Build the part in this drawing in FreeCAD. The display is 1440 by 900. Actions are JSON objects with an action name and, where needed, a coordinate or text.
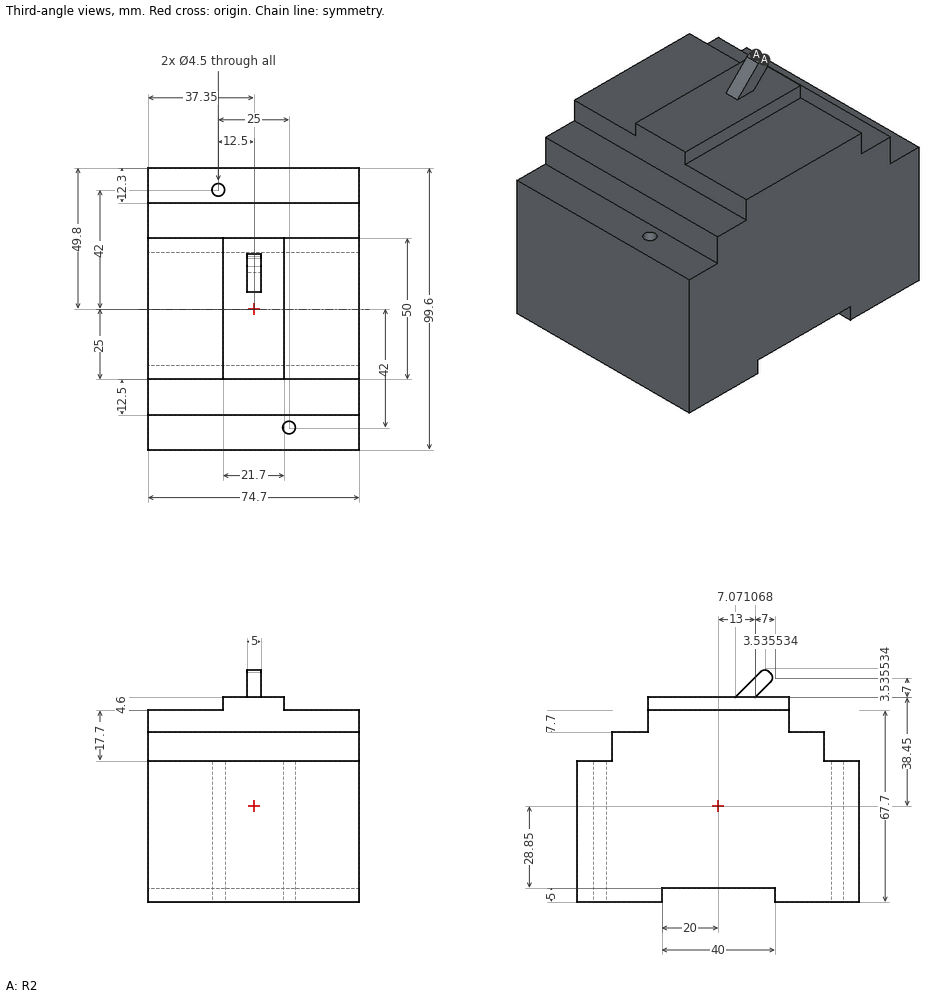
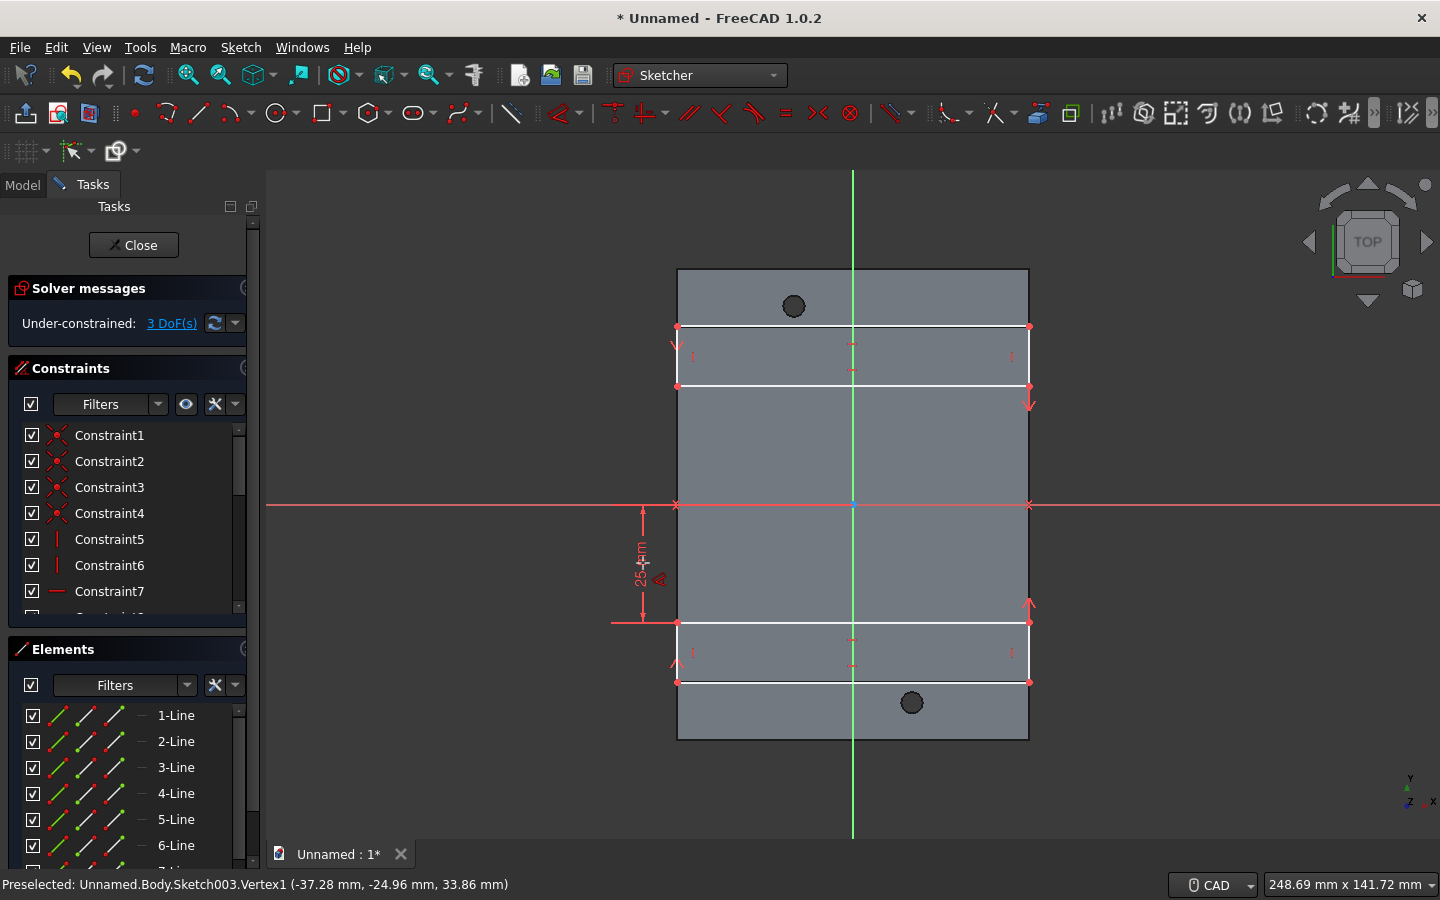
{"action": "left_click", "coordinate": [677, 641]}
{"action": "left_click", "coordinate": [643, 653]}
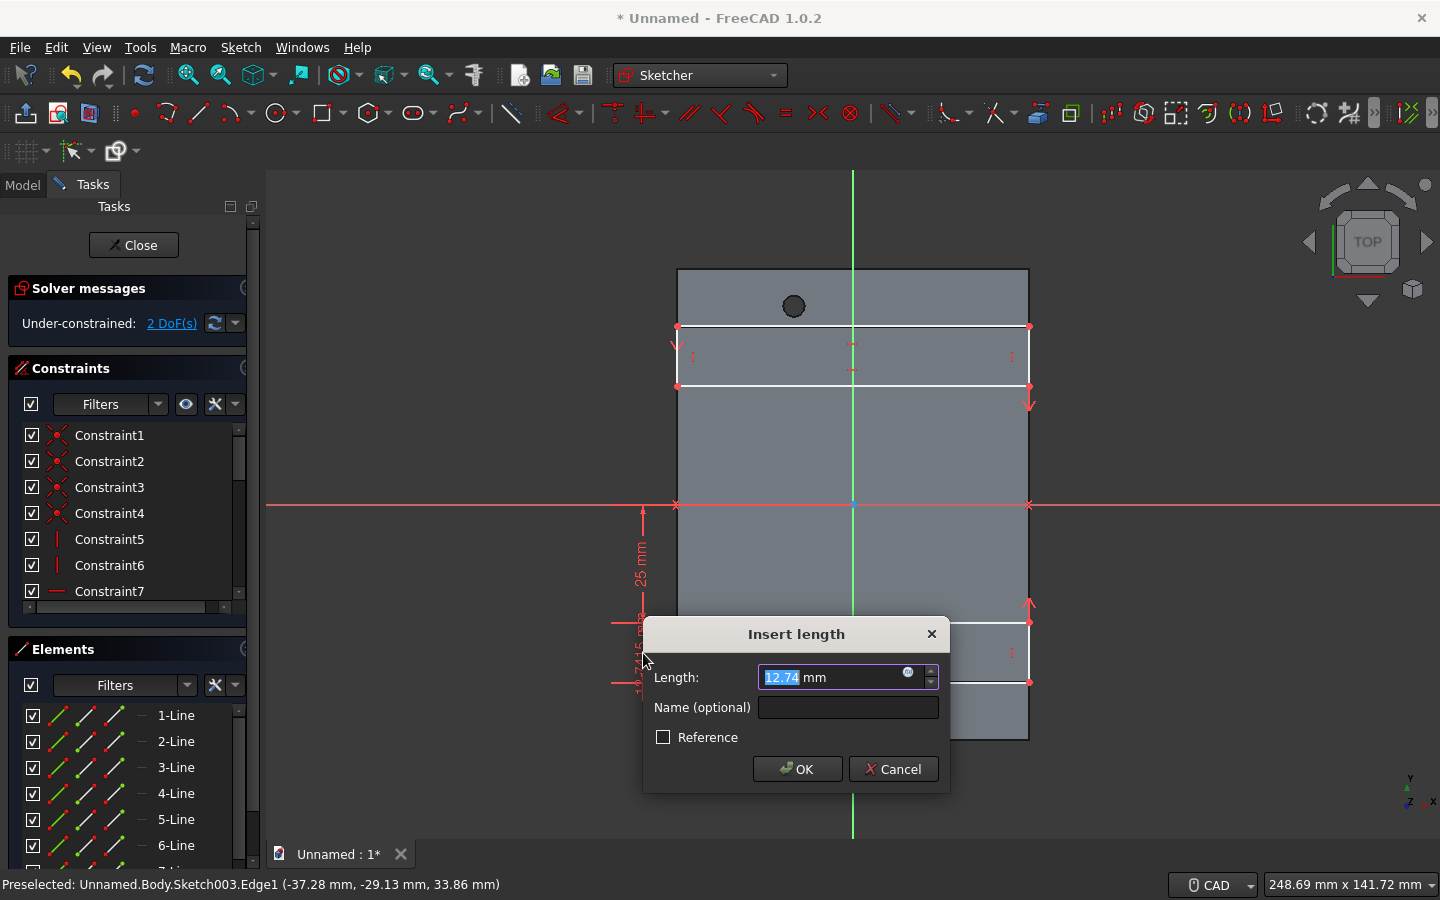
{"action": "type", "text": "12.5"}
{"action": "key", "text": "Return"}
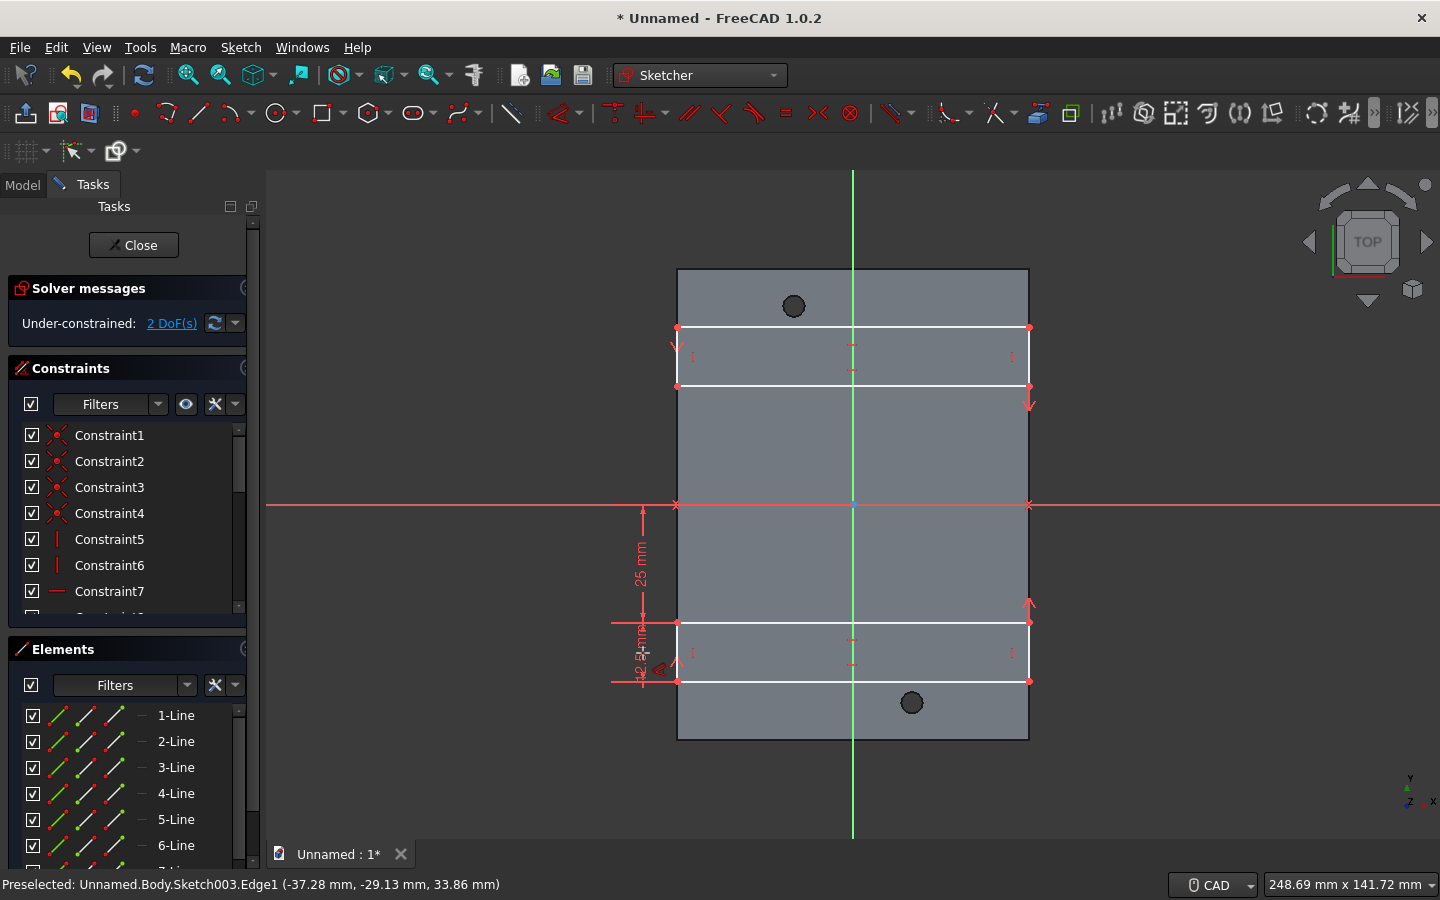
{"action": "left_click", "coordinate": [783, 682]}
{"action": "left_click", "coordinate": [772, 716]}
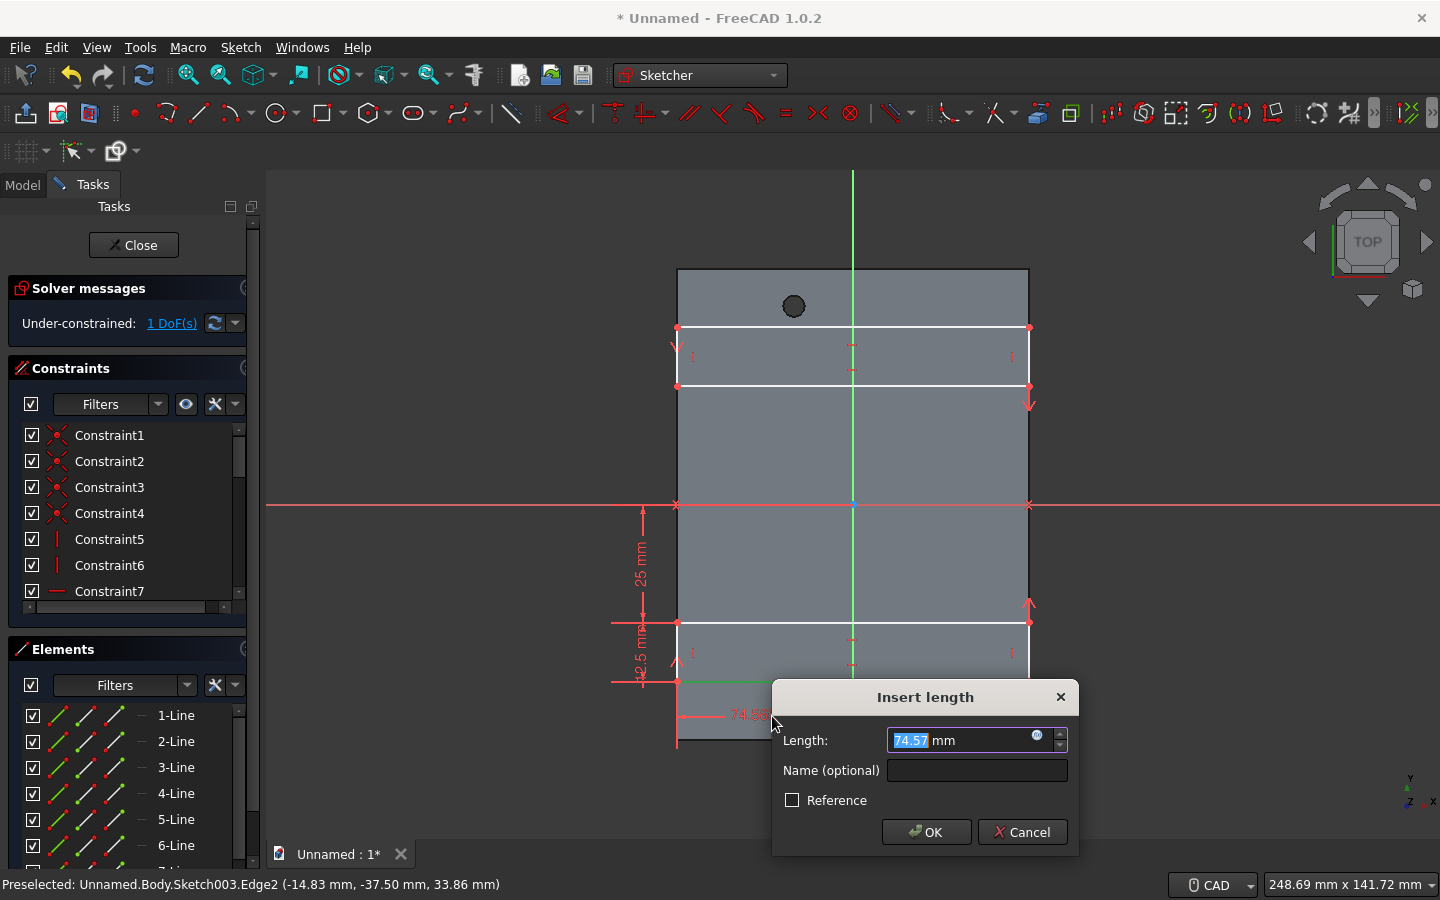
{"action": "type", "text": "74.7"}
{"action": "key", "text": "Return"}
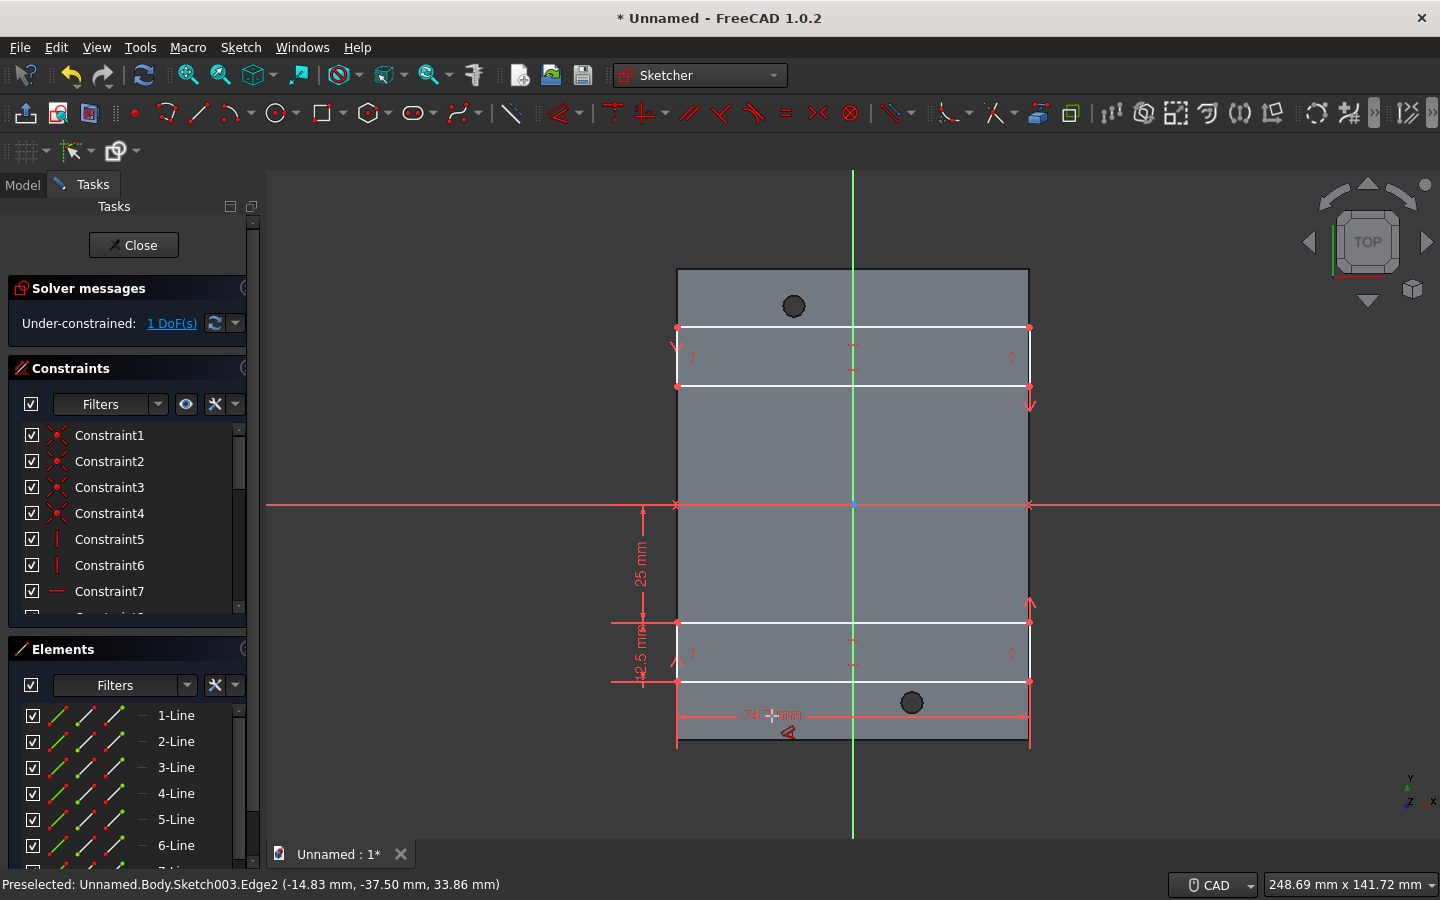
{"action": "left_click", "coordinate": [677, 623]}
{"action": "left_click", "coordinate": [765, 657]}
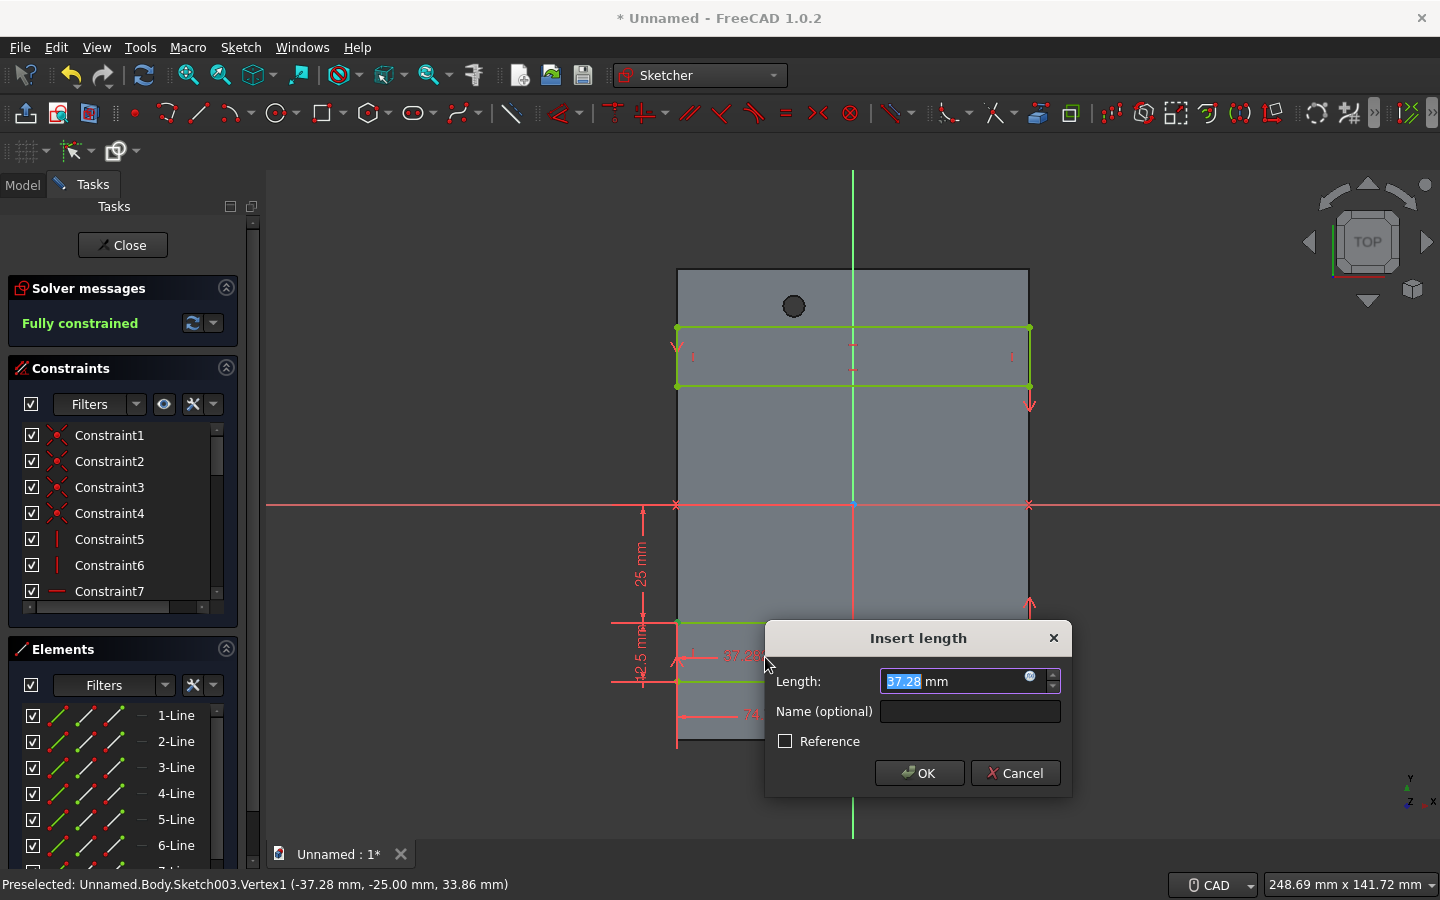
{"action": "type", "text": "37.35"}
{"action": "key", "text": "Return"}
{"action": "key", "text": "Escape"}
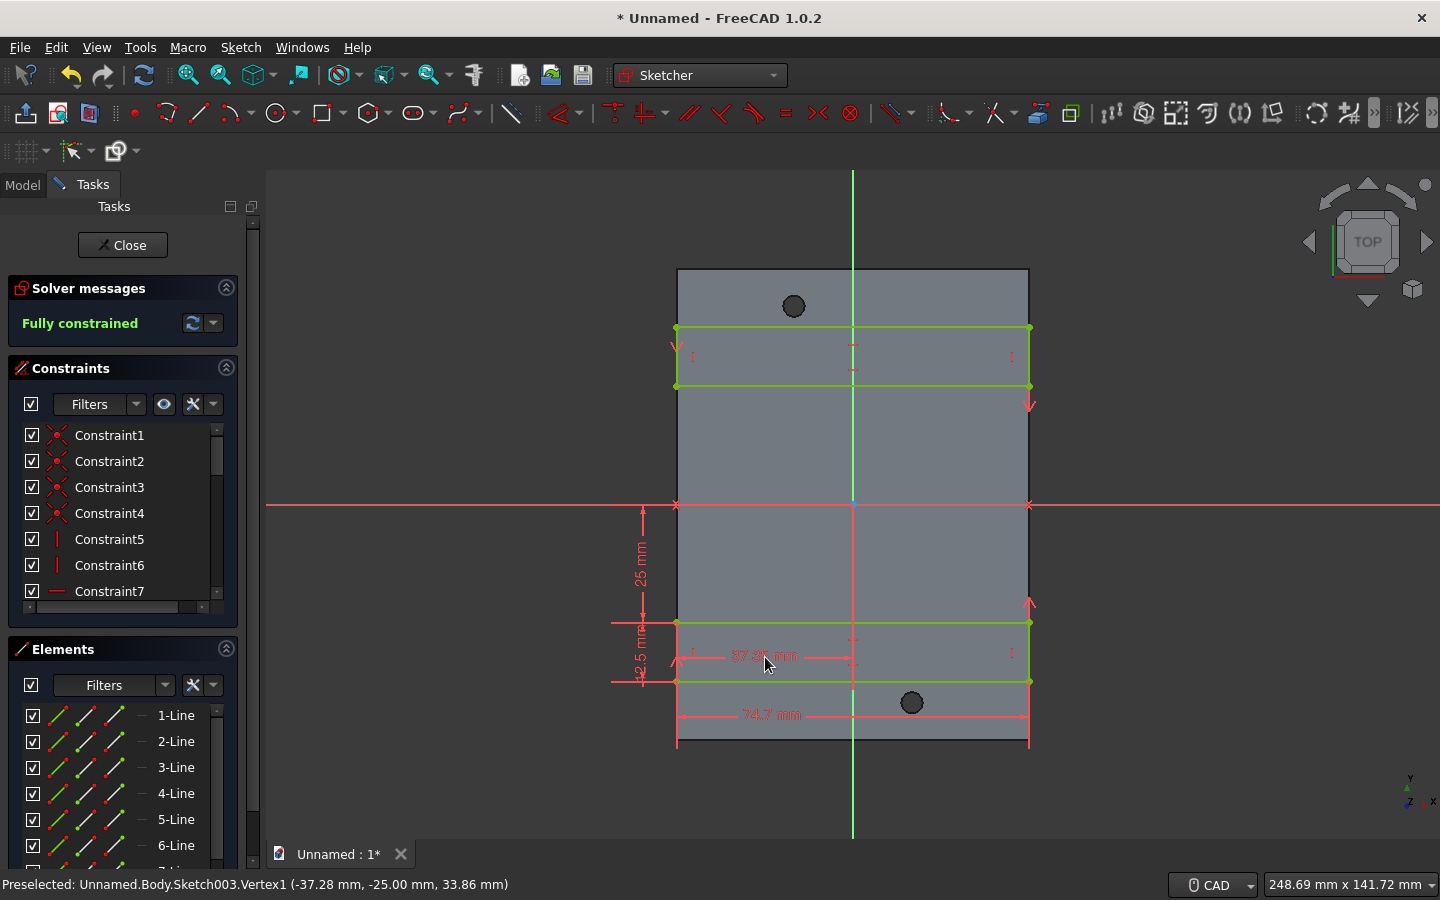
{"action": "left_click", "coordinate": [123, 245]}